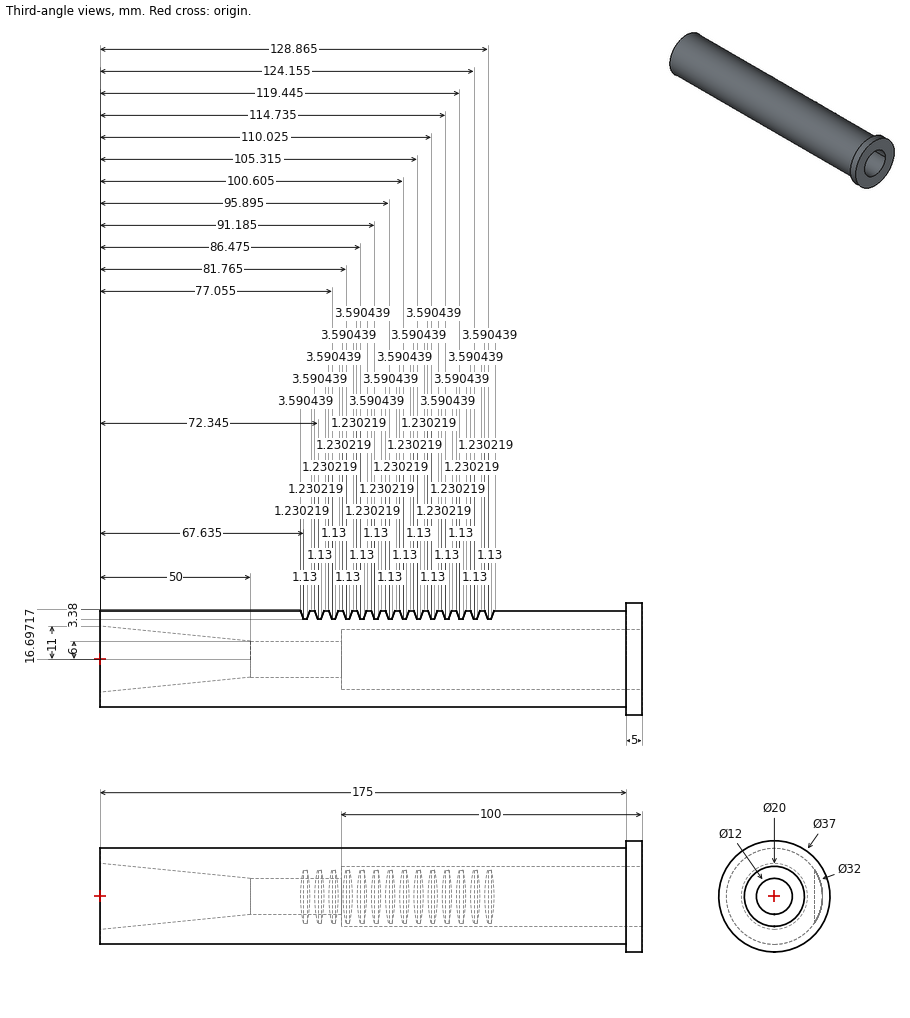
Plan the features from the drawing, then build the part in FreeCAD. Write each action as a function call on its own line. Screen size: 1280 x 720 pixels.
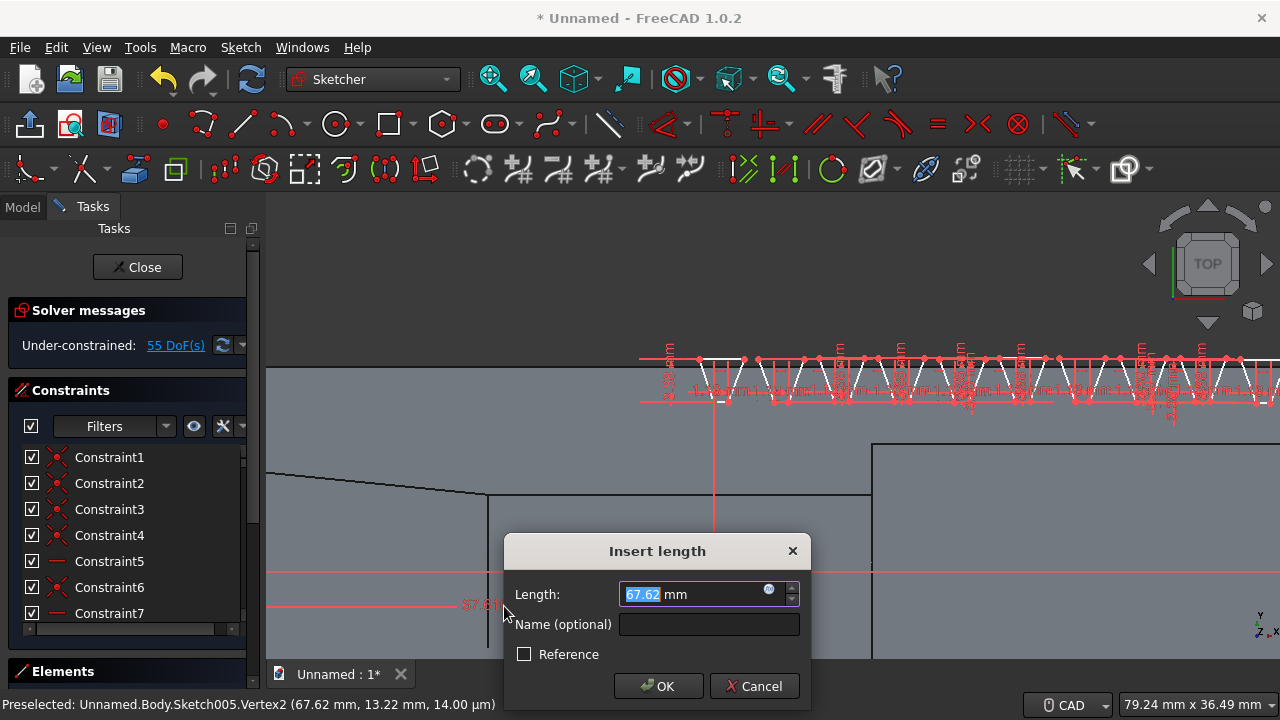
text(67.635)
key(Return)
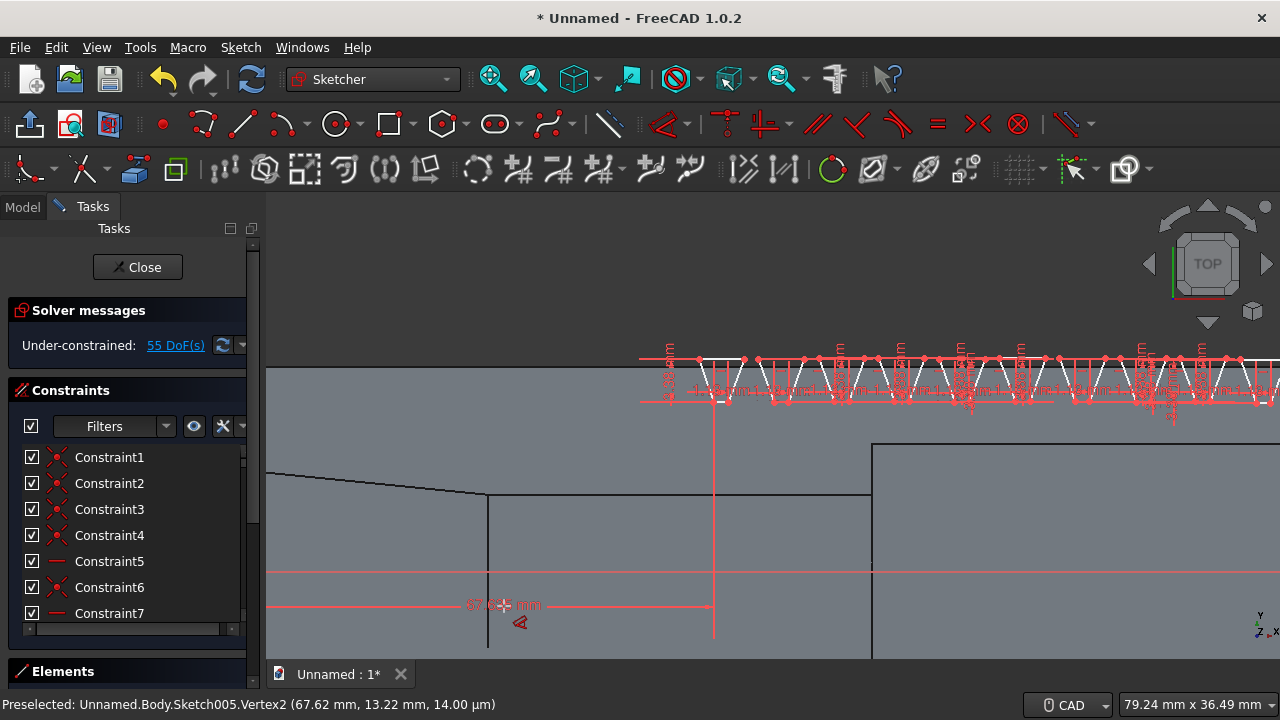
click(774, 402)
click(424, 606)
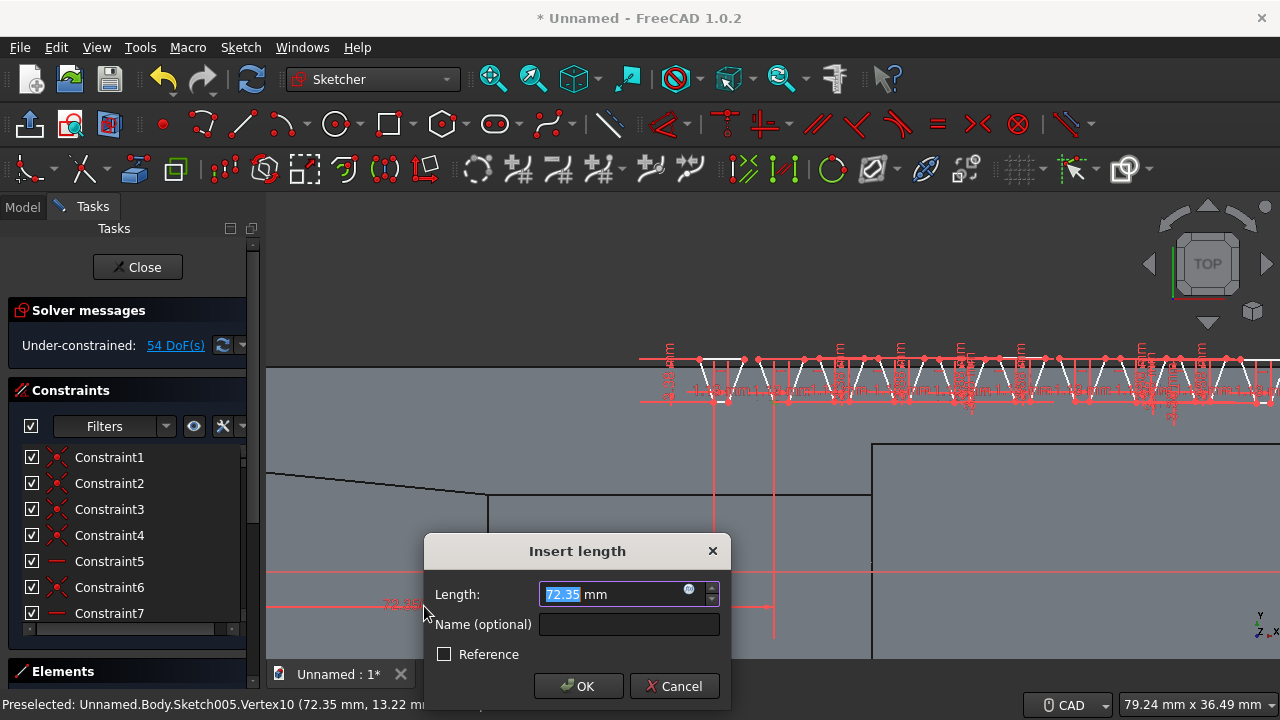
text(72.345)
key(Return)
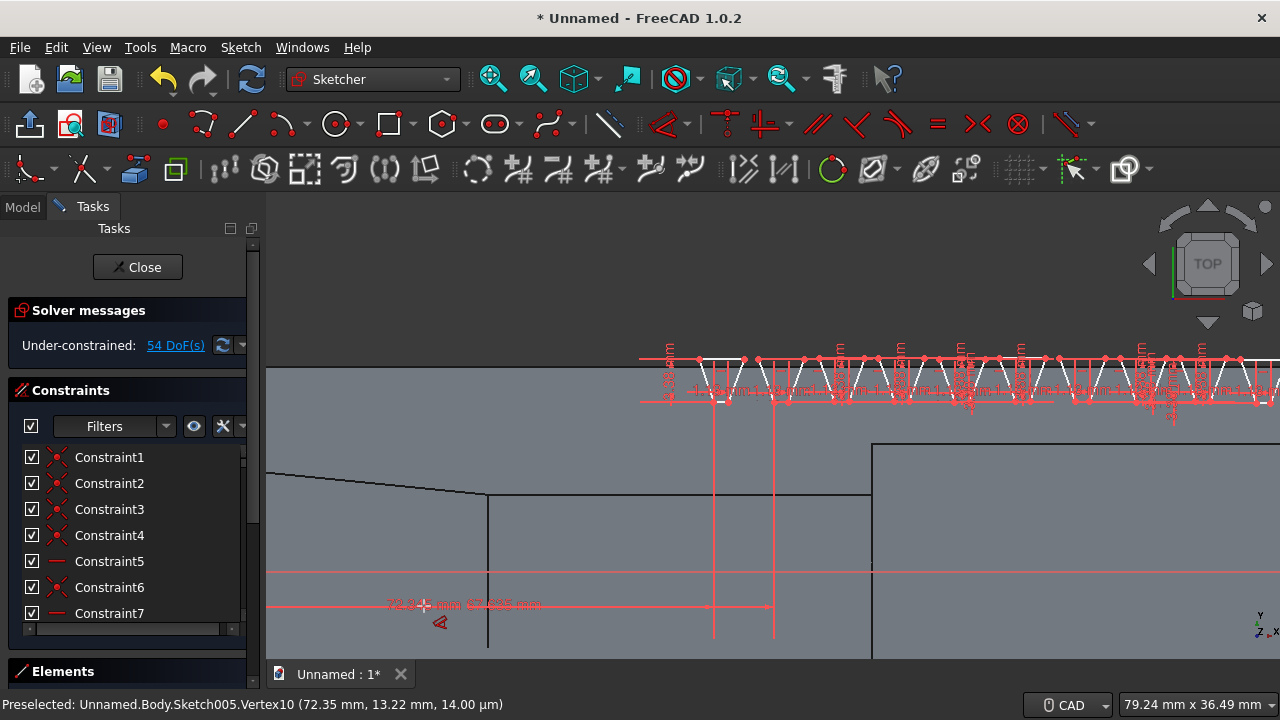
click(835, 402)
click(689, 606)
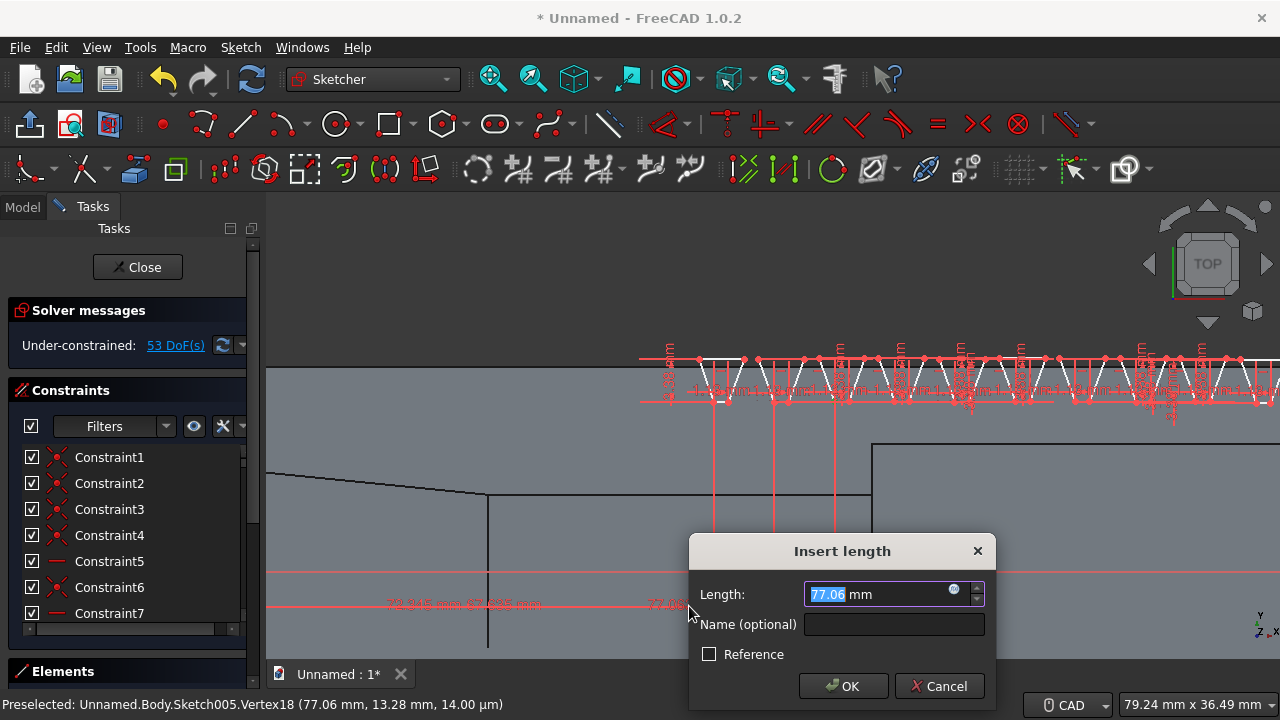
text(77.055)
key(Return)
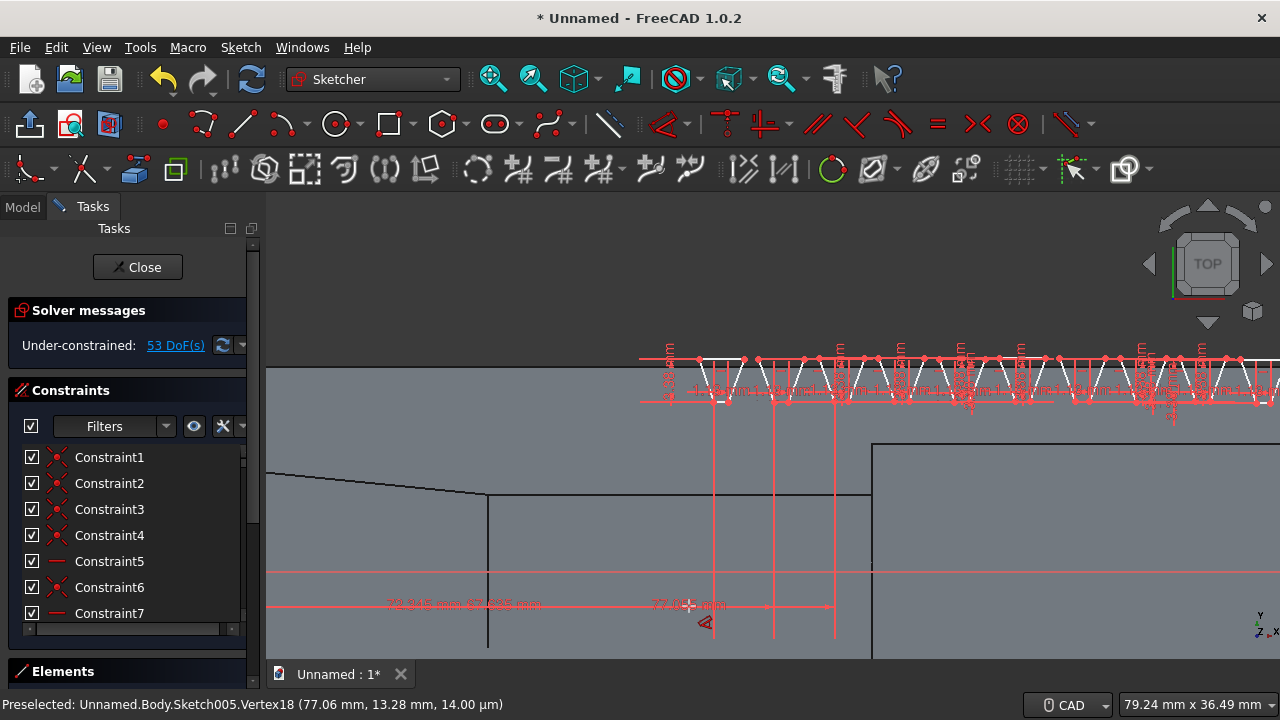
click(895, 402)
click(594, 606)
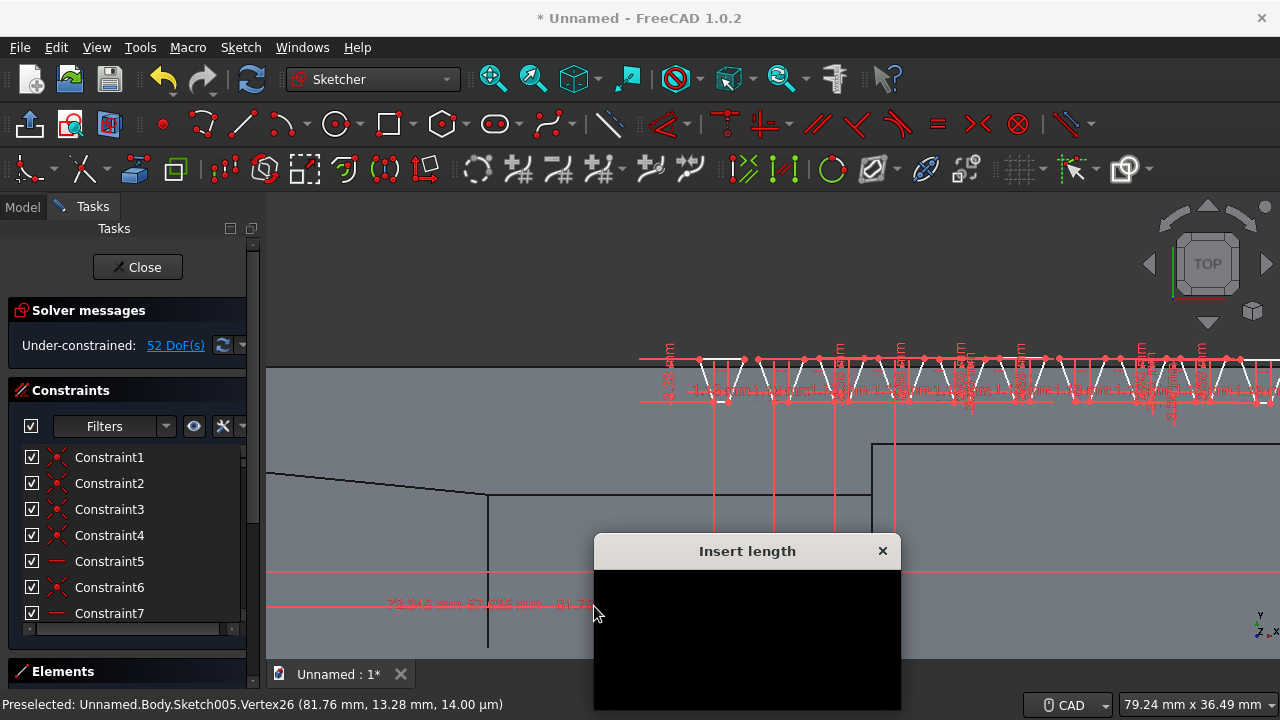
text(81.765)
key(Return)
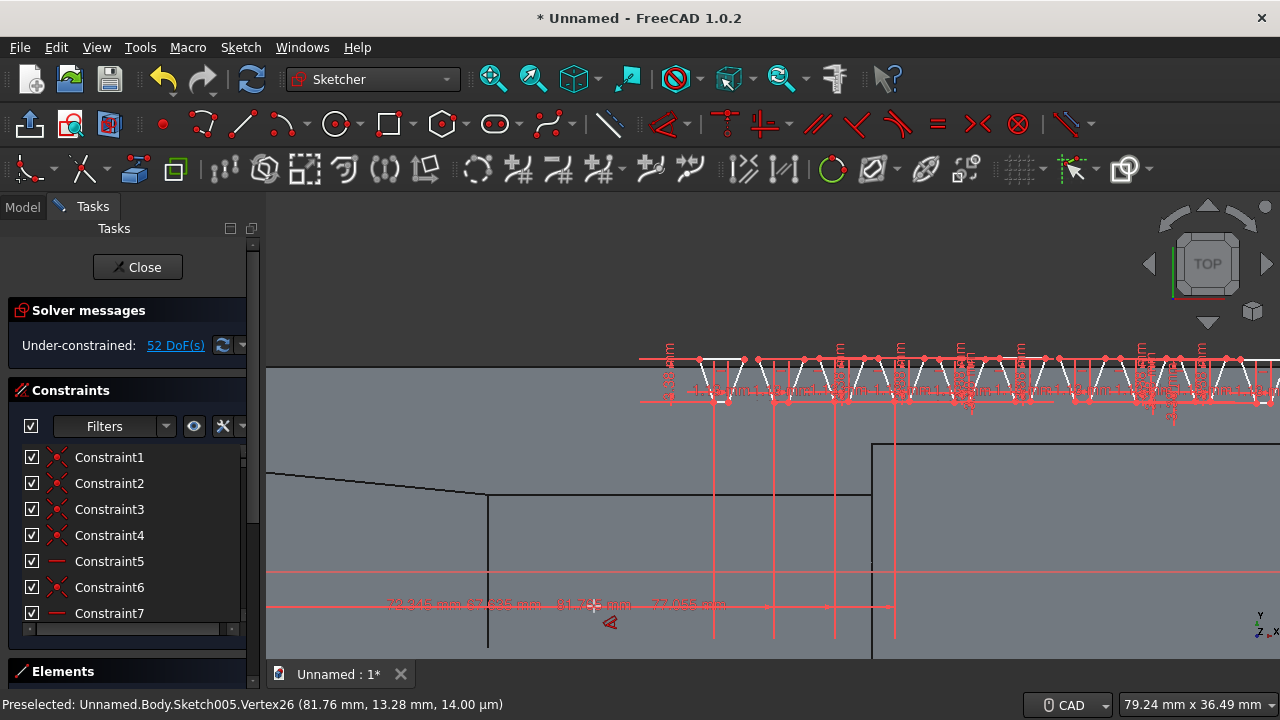
click(955, 402)
click(777, 606)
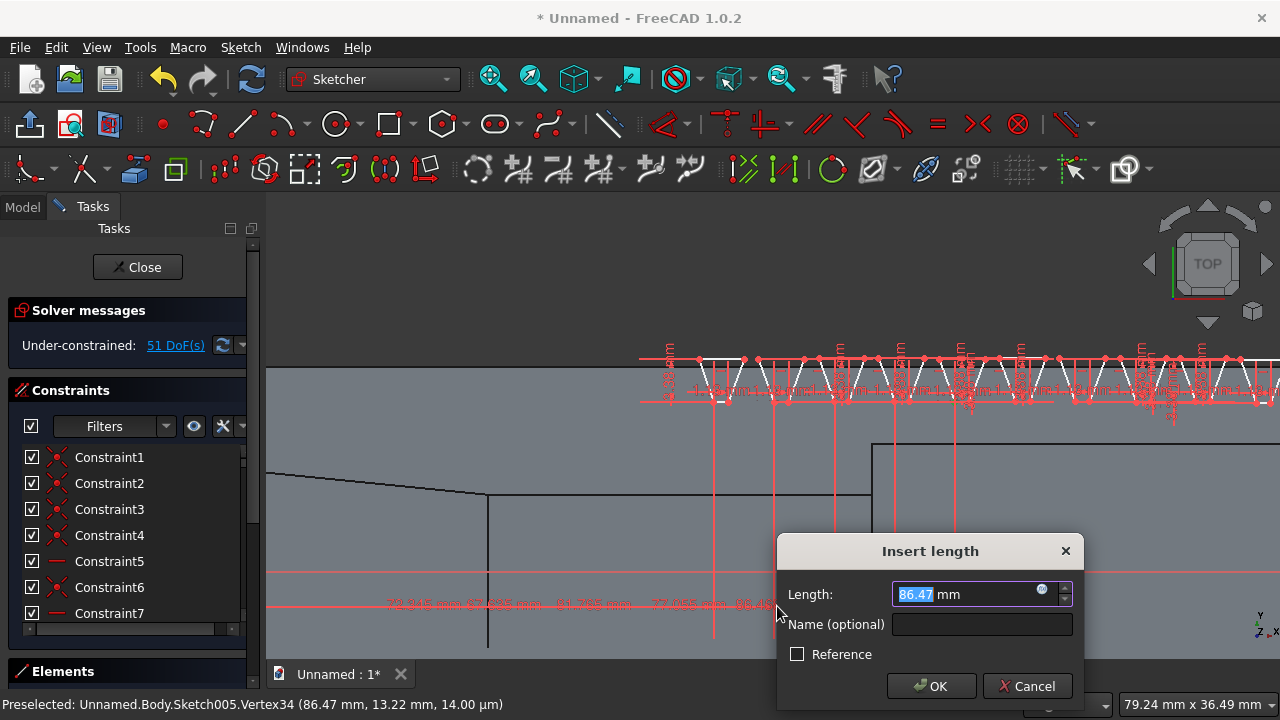
text(86.475)
key(Return)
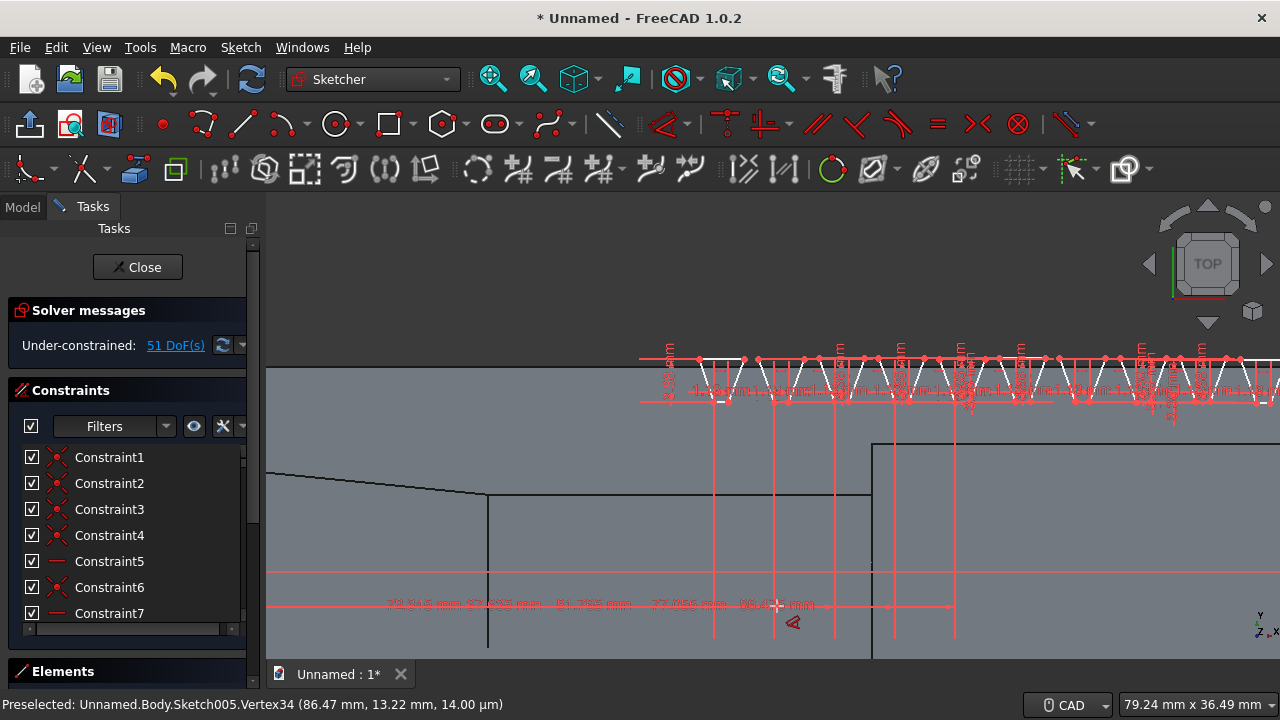
click(1016, 402)
click(907, 606)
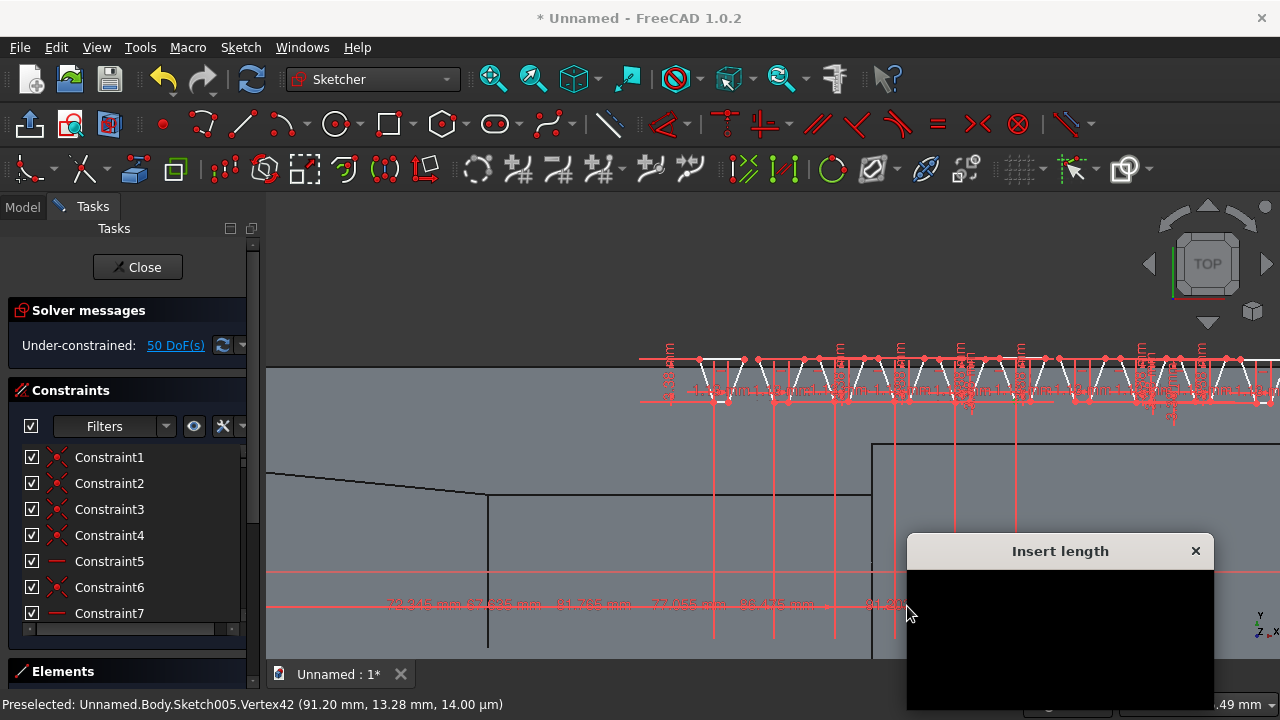
text(91.185)
key(Return)